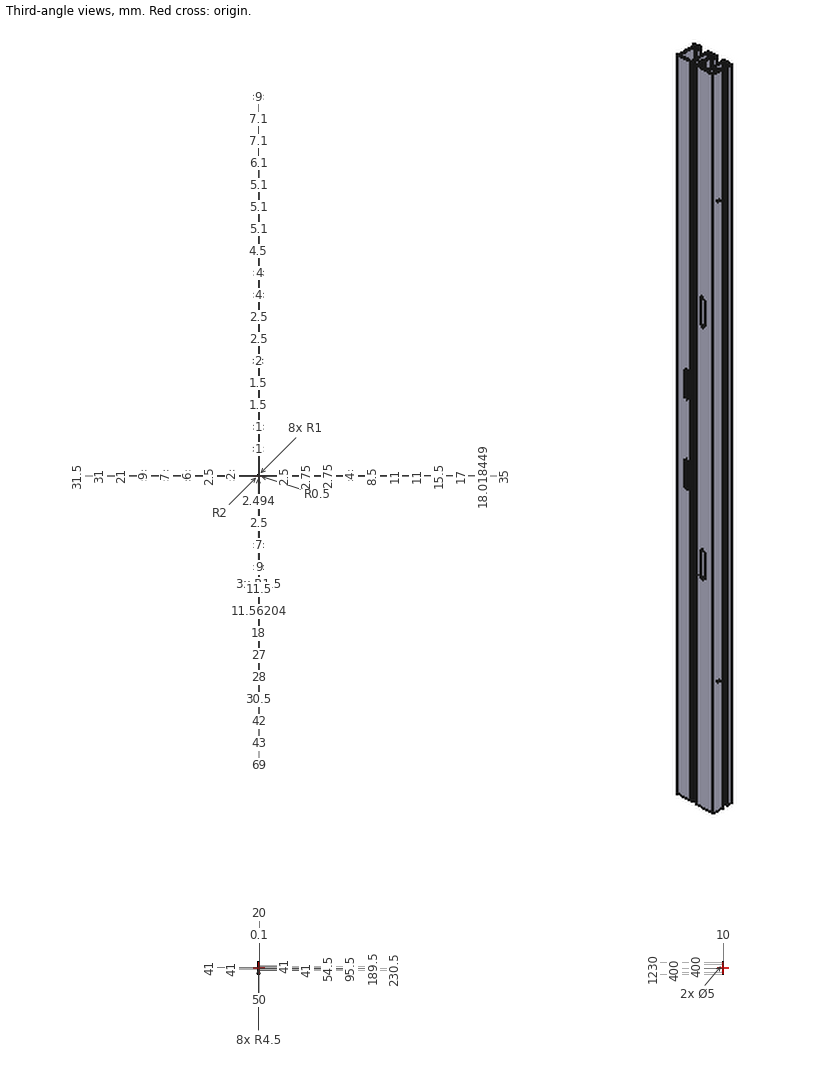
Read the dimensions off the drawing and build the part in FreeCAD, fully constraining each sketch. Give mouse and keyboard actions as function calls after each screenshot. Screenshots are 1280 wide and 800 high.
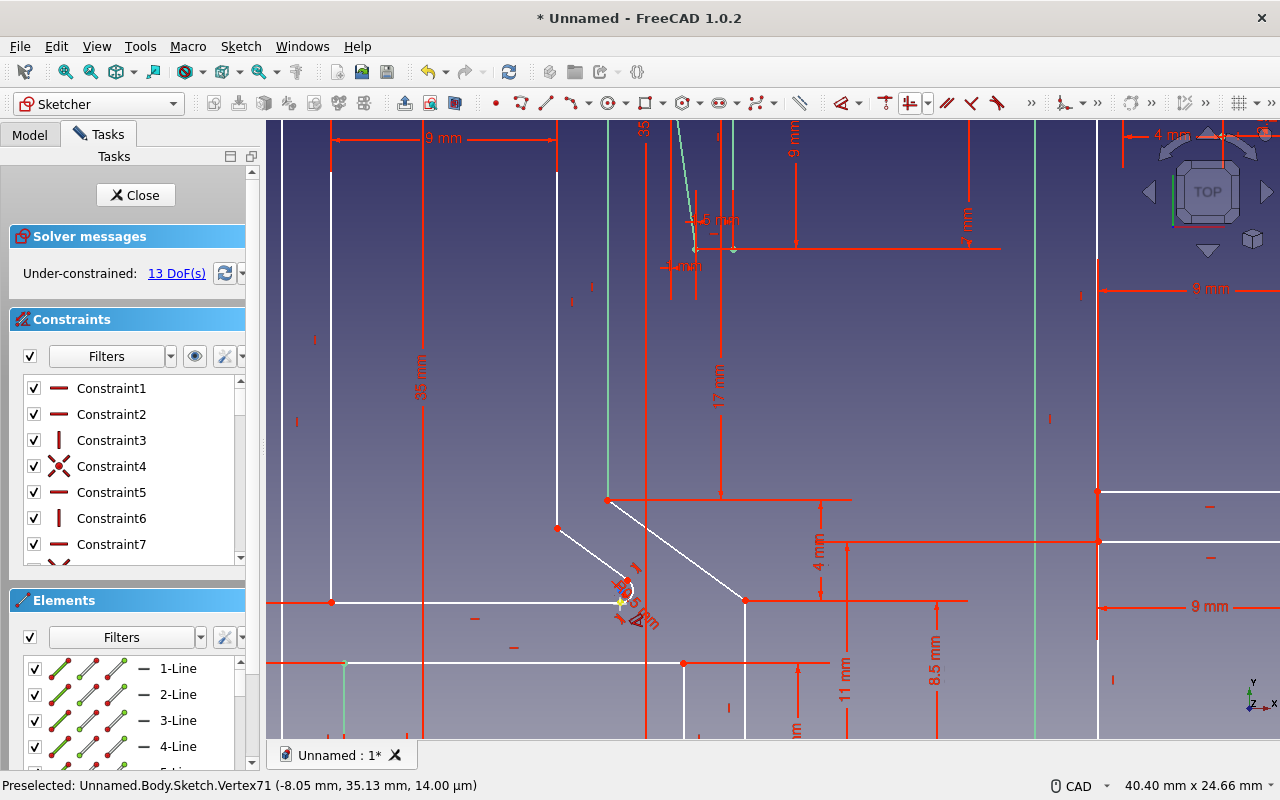
click(620, 603)
click(586, 632)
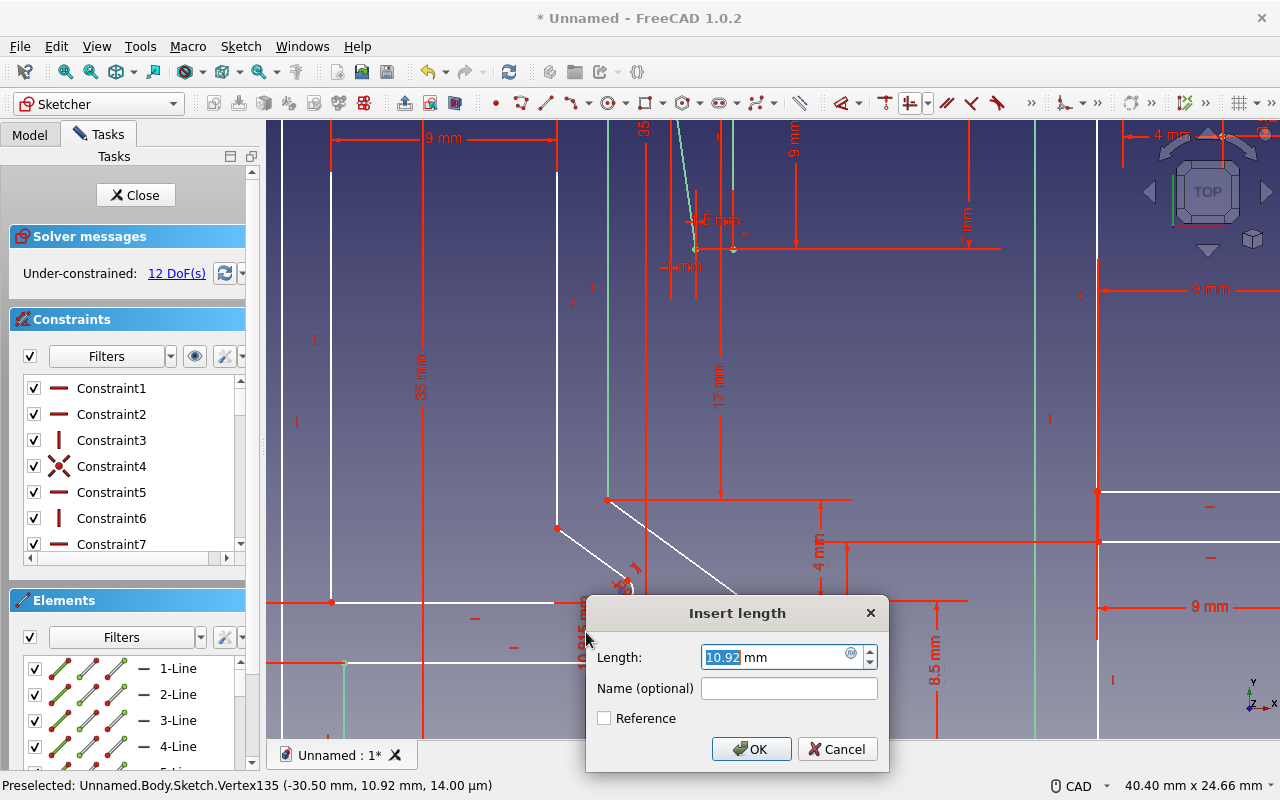
text(11)
key(Return)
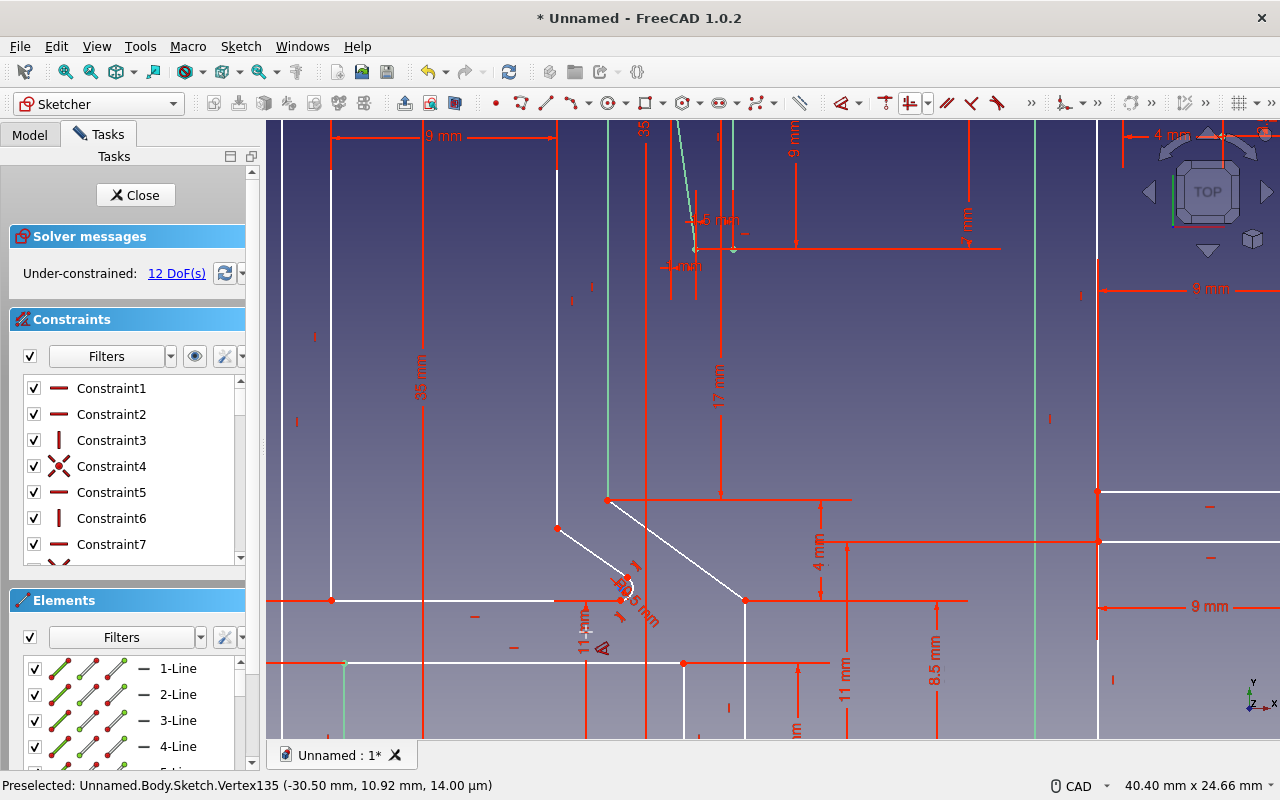
scroll(789, 426, down, 6)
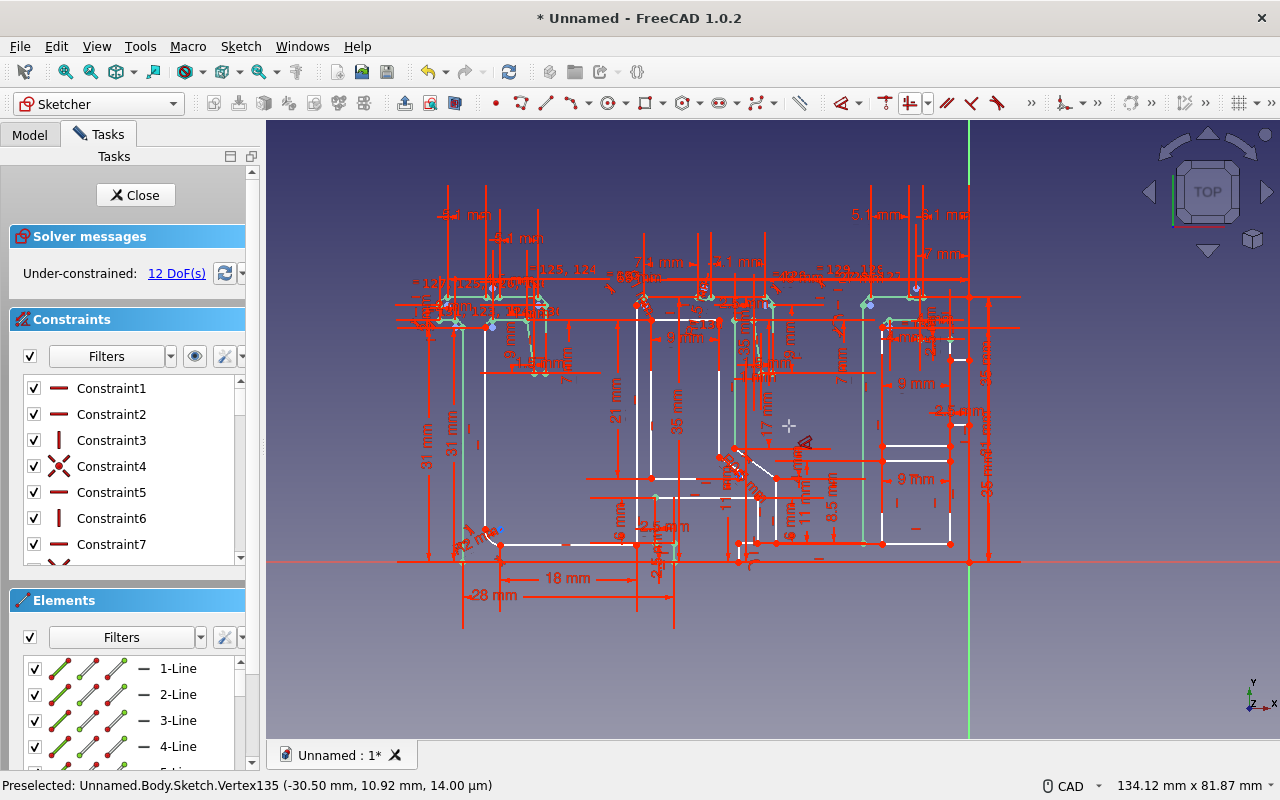
click(651, 479)
click(810, 596)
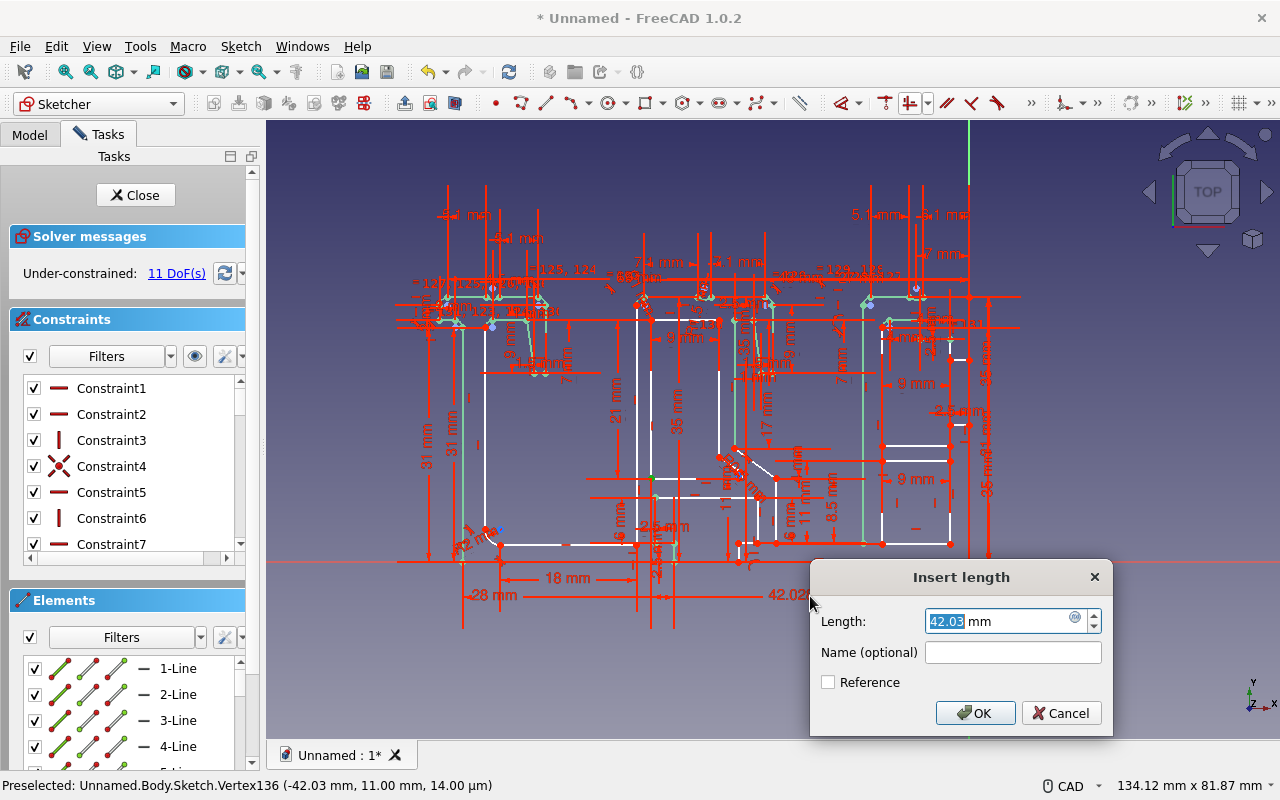
text(42)
key(Return)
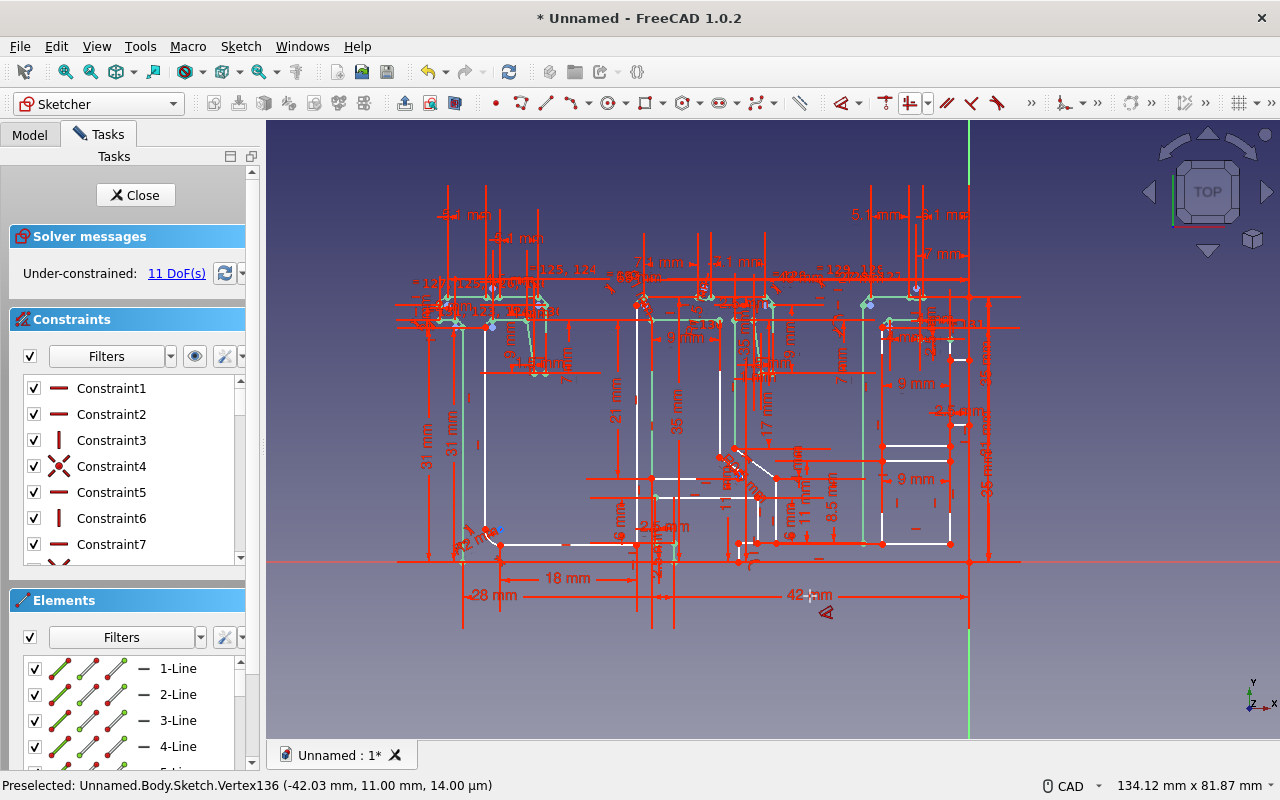
click(637, 377)
click(603, 425)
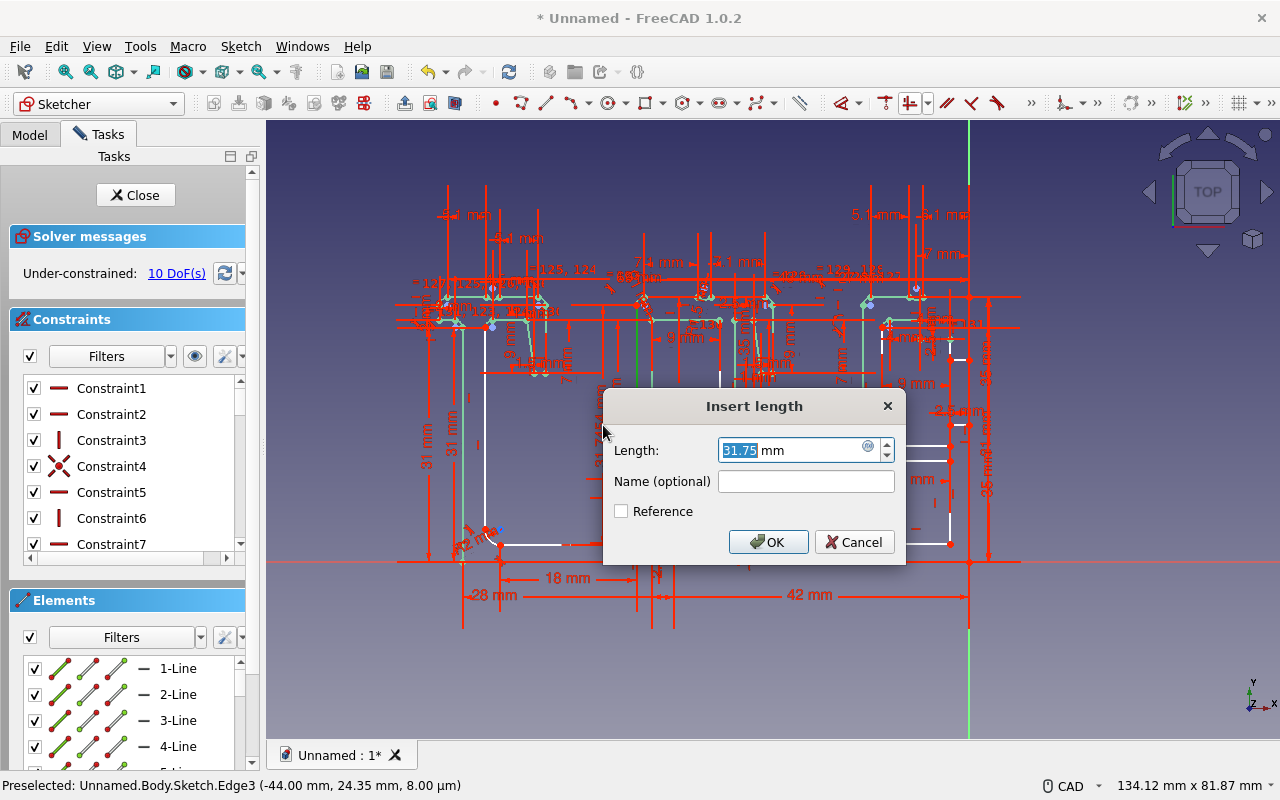
text(31.5)
key(Return)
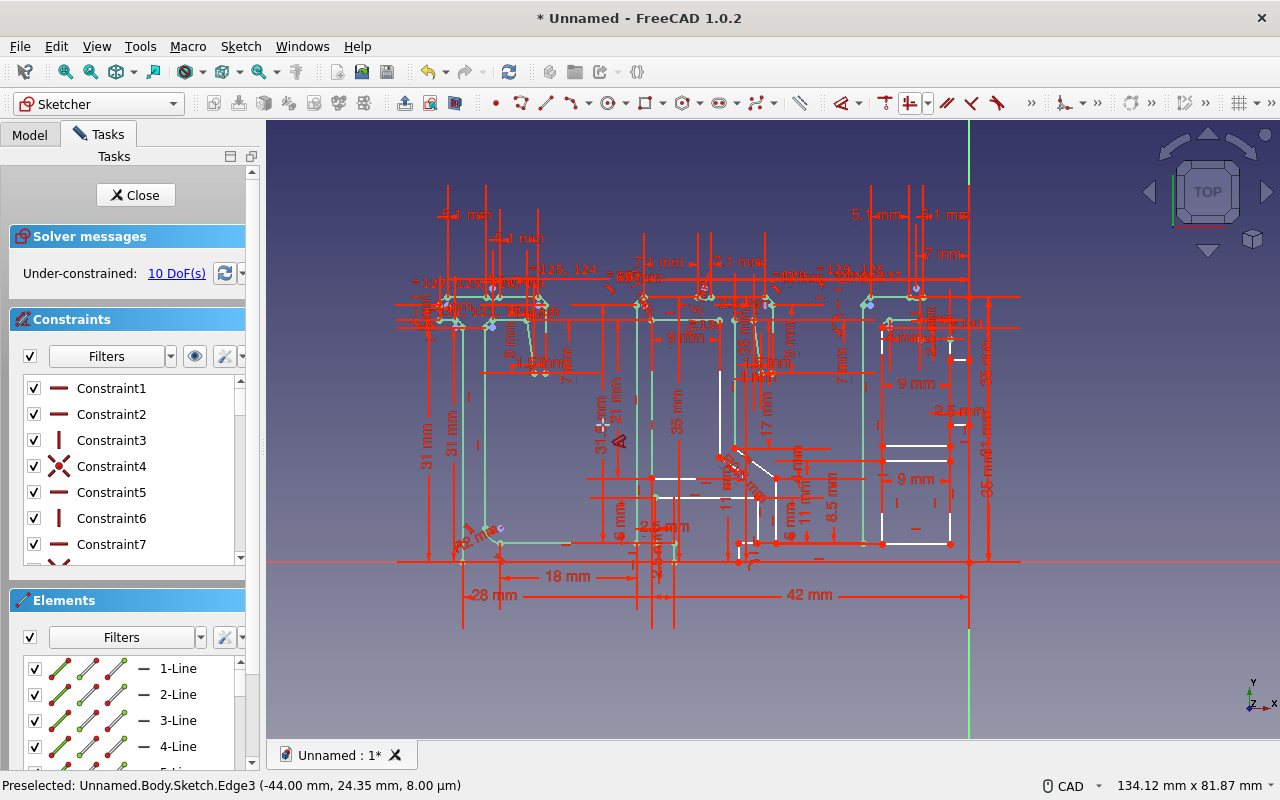
click(808, 562)
click(907, 596)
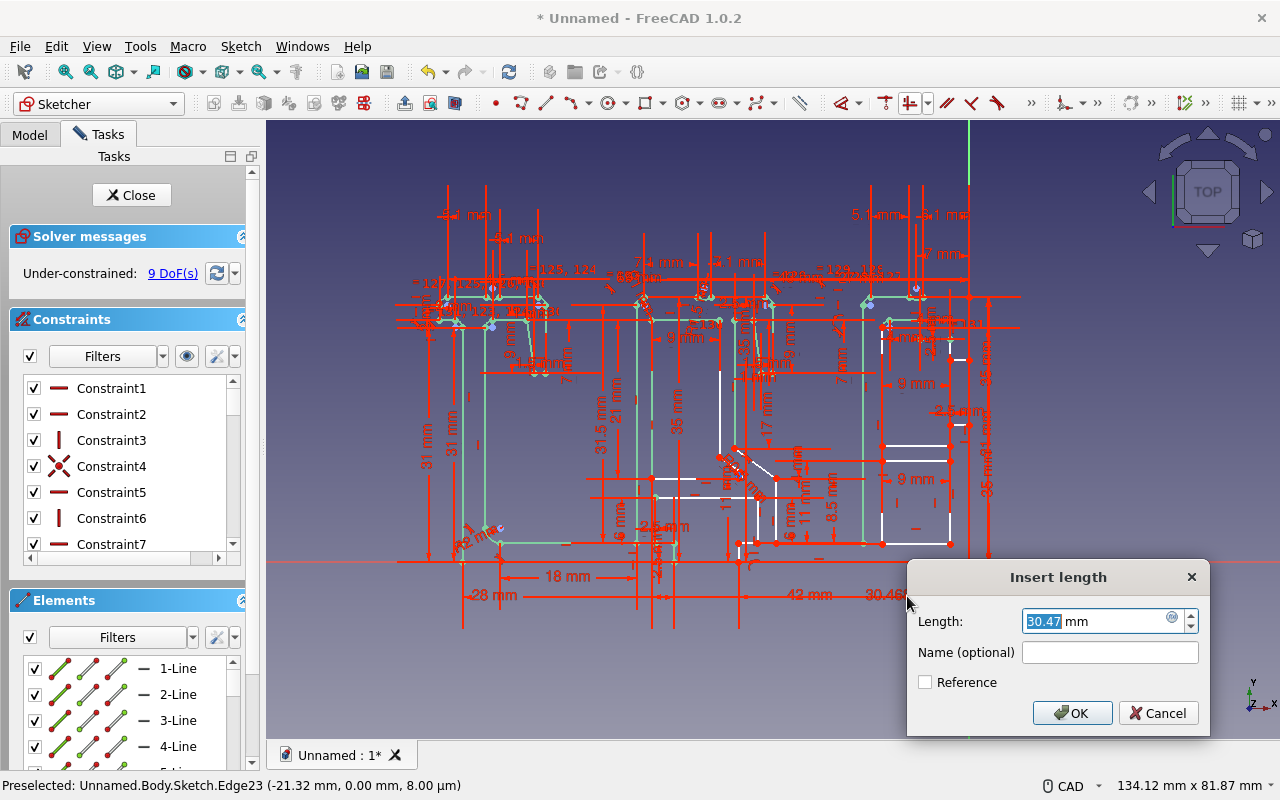
text(30.5)
key(Return)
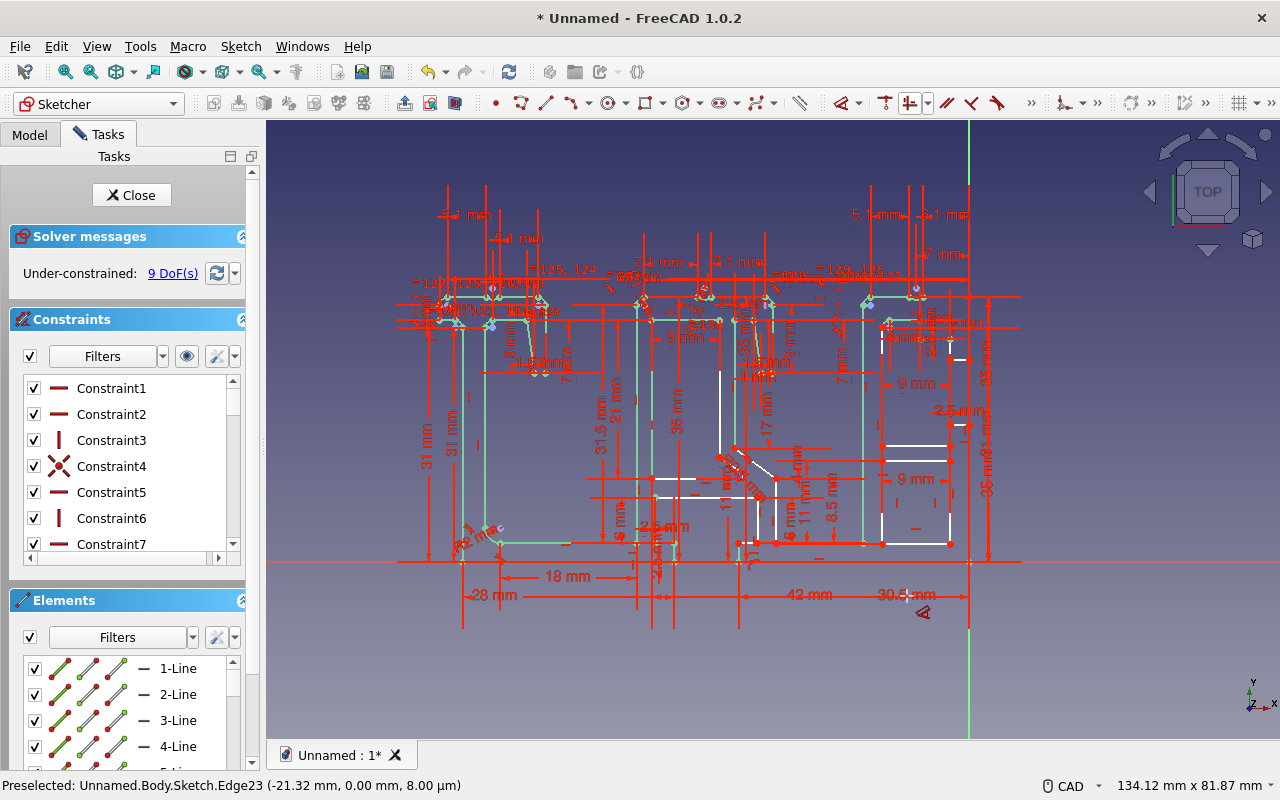
scroll(950, 436, up, 4)